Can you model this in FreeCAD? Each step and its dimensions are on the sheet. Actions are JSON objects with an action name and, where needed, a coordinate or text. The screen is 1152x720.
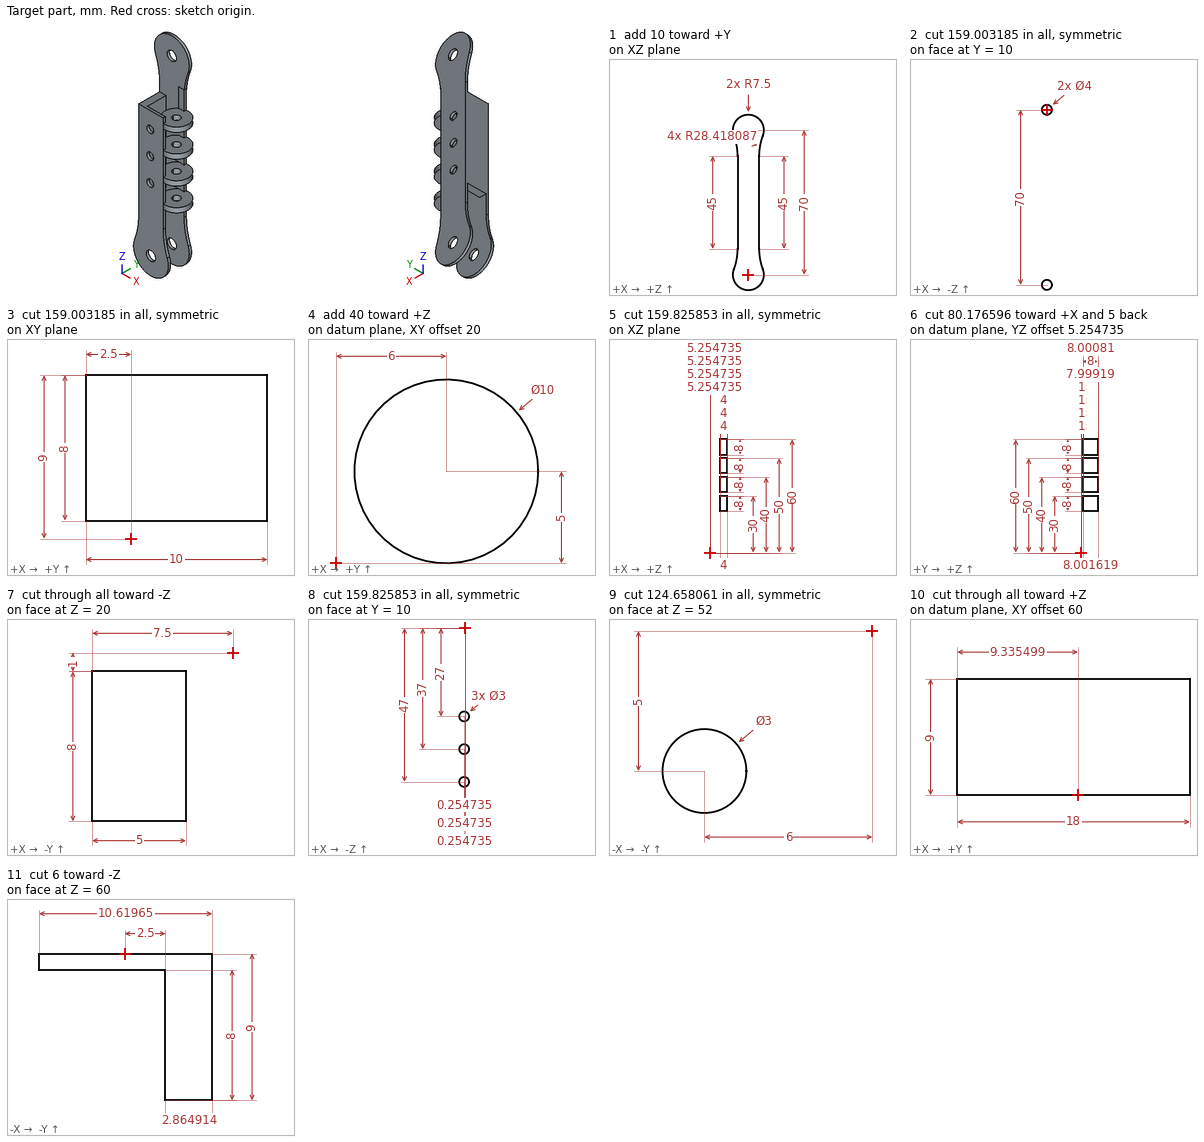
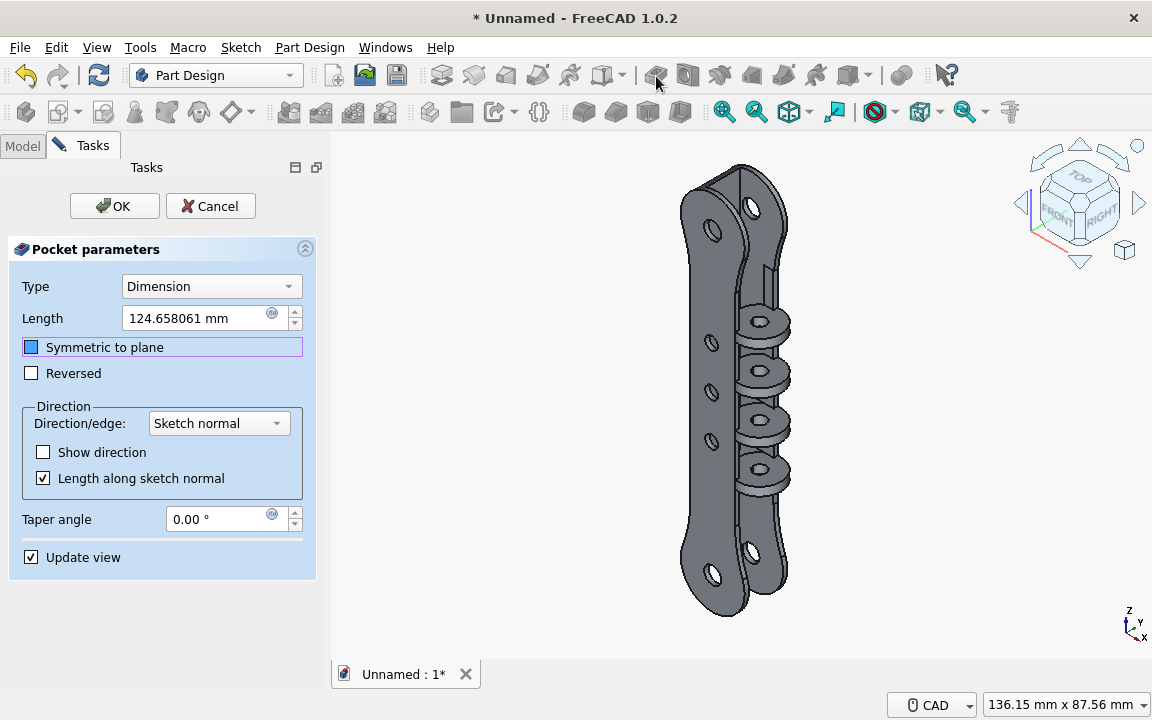
{"action": "left_click", "coordinate": [30, 347]}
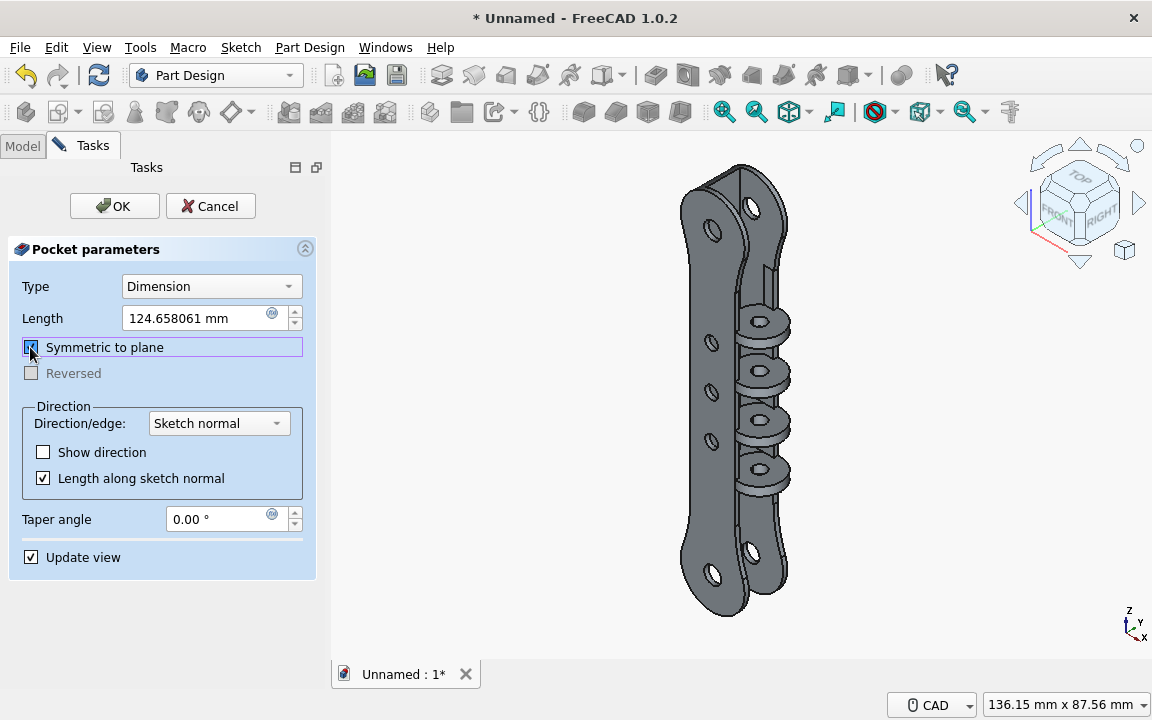
{"action": "left_click", "coordinate": [115, 206]}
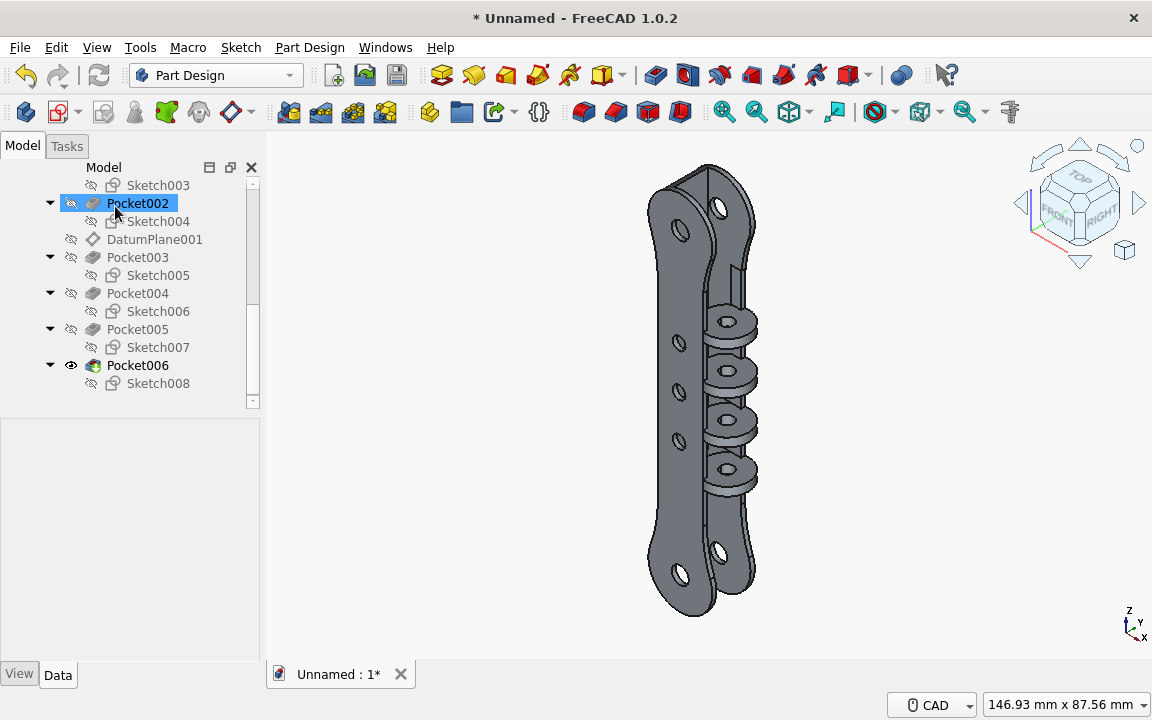
{"action": "scroll", "coordinate": [740, 269], "scroll_direction": "up", "scroll_amount": 15}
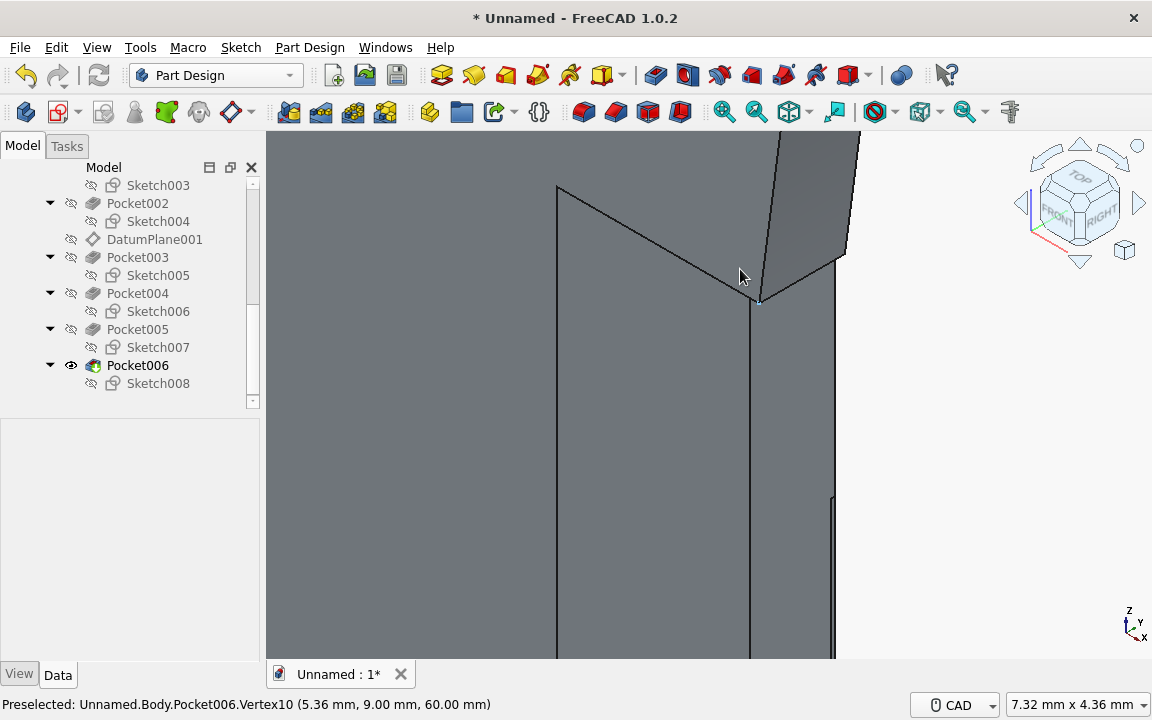
{"action": "scroll", "coordinate": [736, 289], "scroll_direction": "up", "scroll_amount": 15}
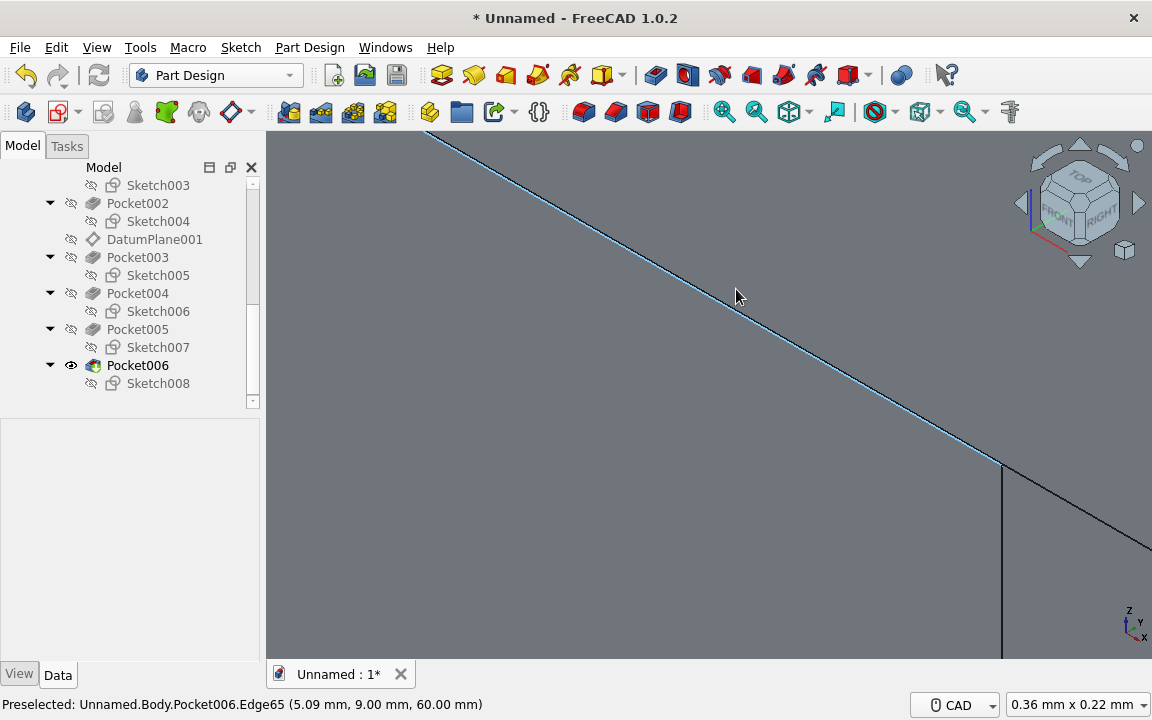
{"action": "left_click", "coordinate": [726, 112]}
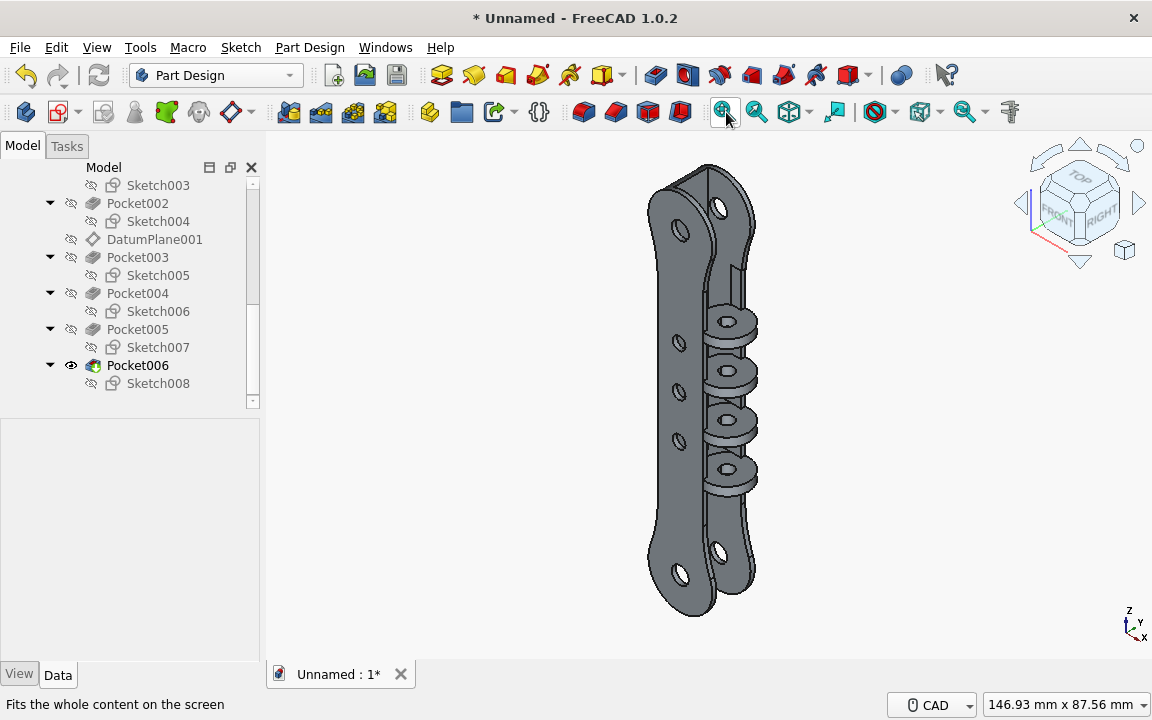
{"action": "key", "text": "2"}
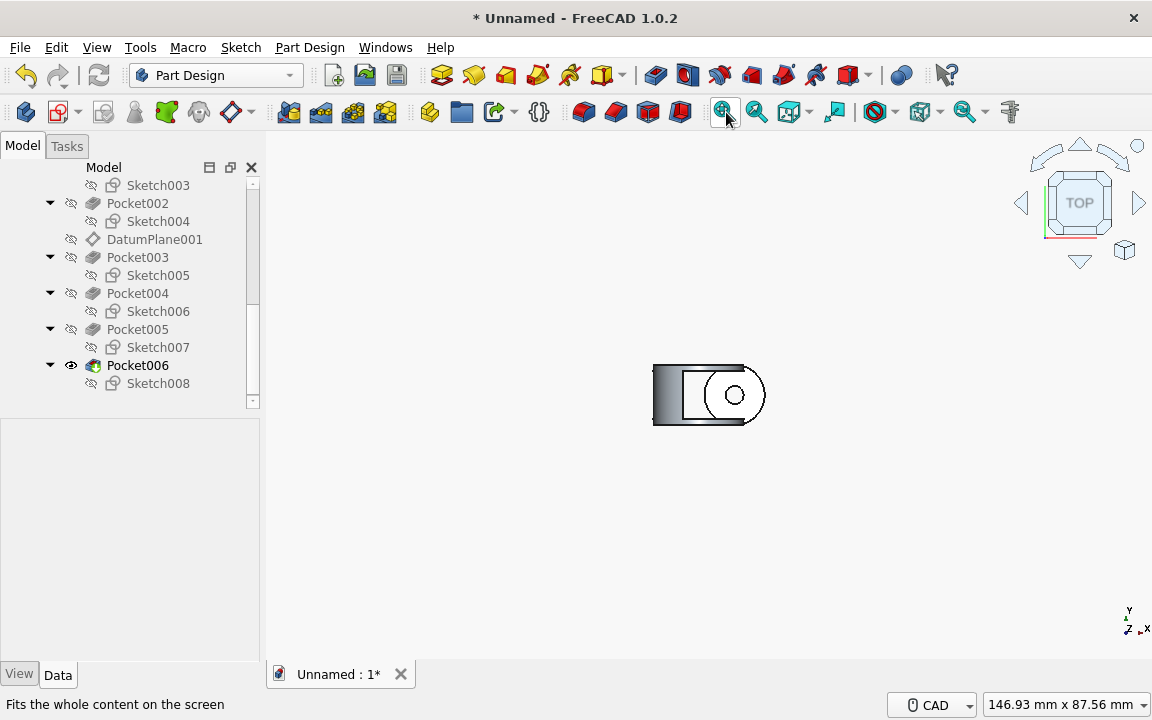
{"action": "left_click", "coordinate": [726, 112]}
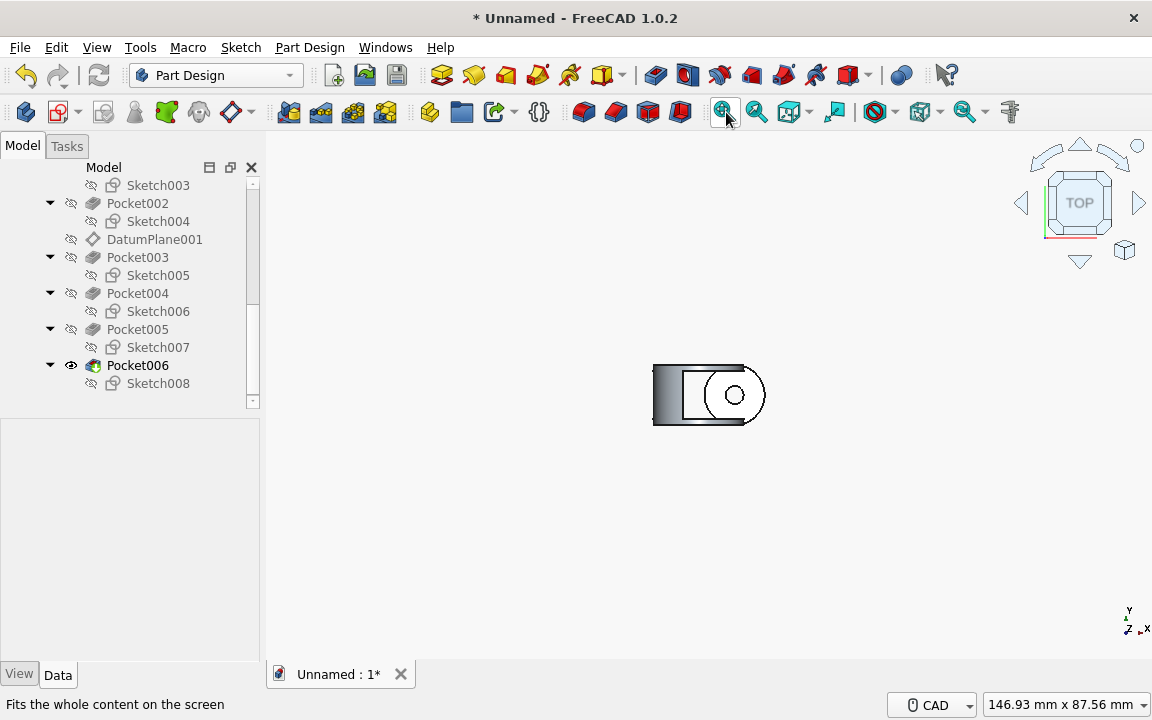
{"action": "scroll", "coordinate": [729, 370], "scroll_direction": "up", "scroll_amount": 15}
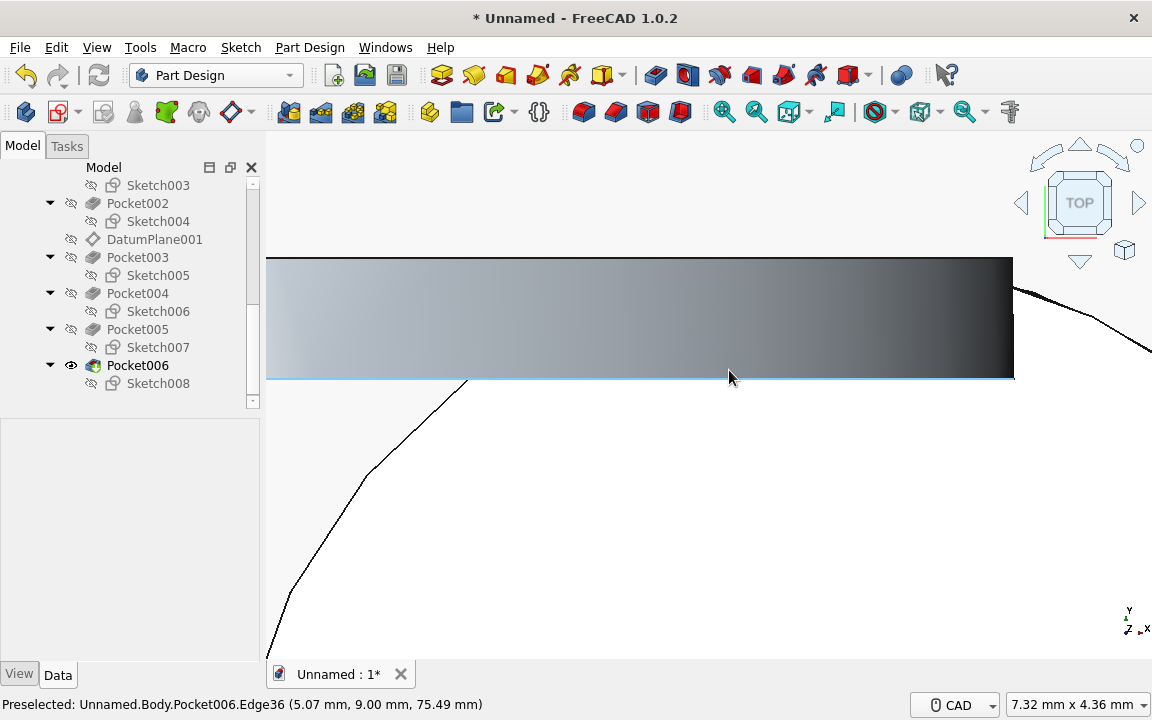
{"action": "scroll", "coordinate": [722, 378], "scroll_direction": "up", "scroll_amount": 15}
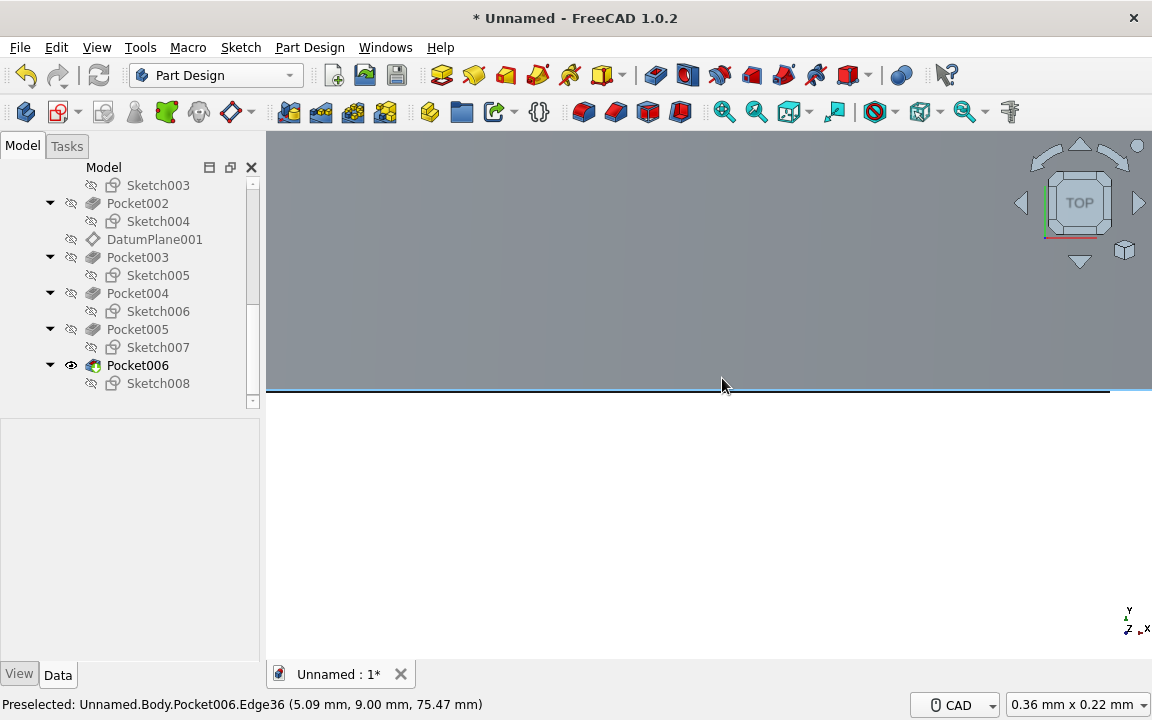
{"action": "left_click", "coordinate": [726, 112]}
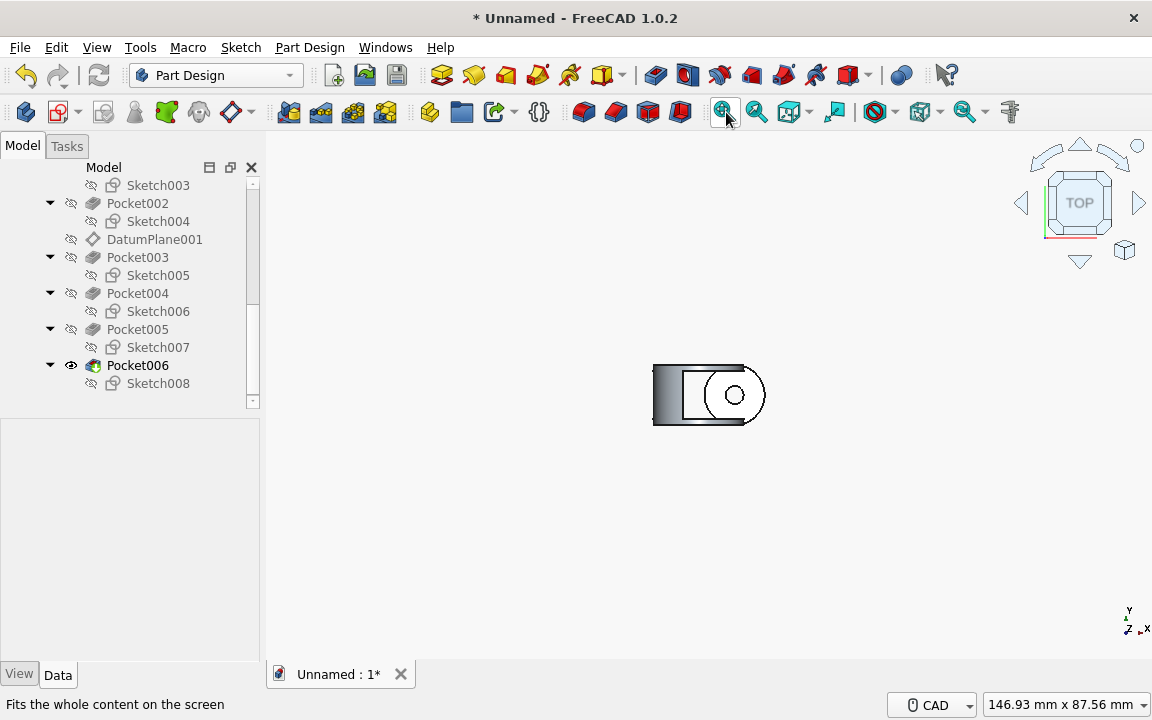
{"action": "key", "text": "0"}